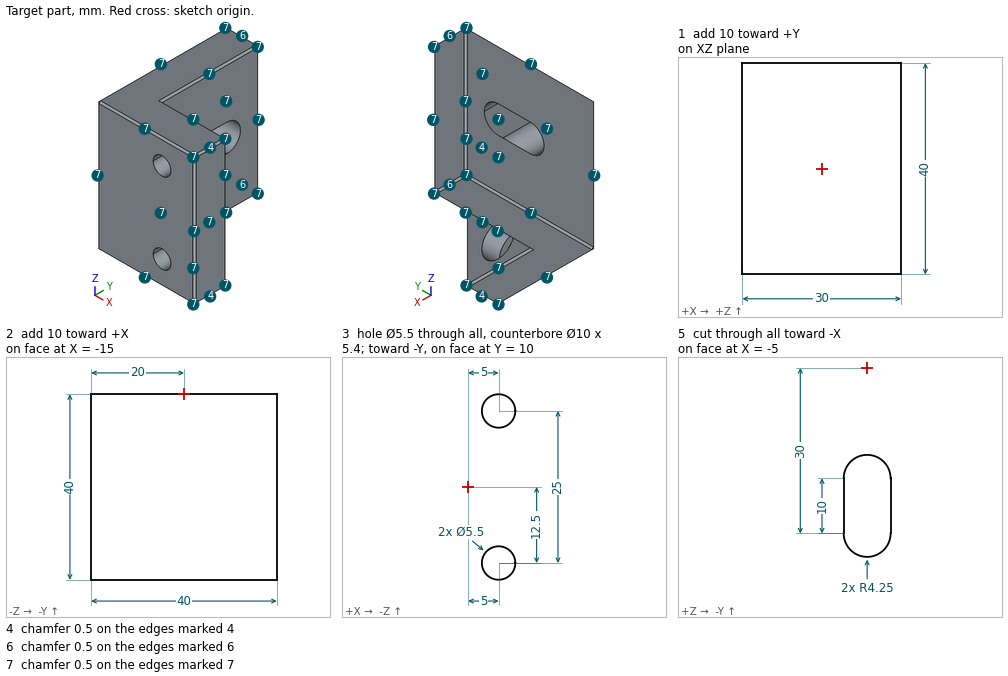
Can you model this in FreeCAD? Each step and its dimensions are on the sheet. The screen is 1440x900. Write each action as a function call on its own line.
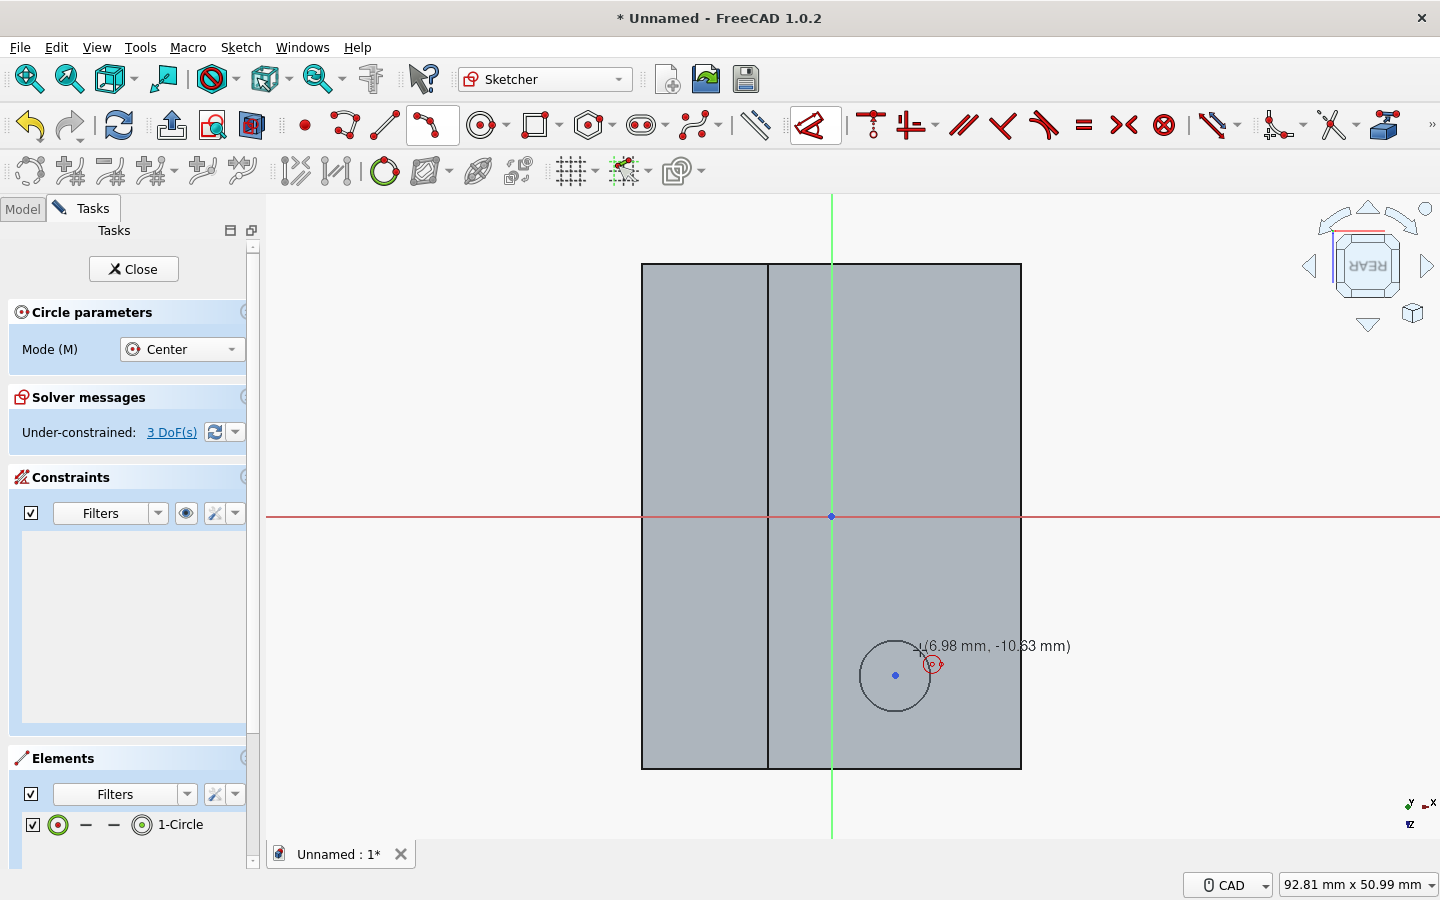
click(895, 358)
click(920, 334)
key(Escape)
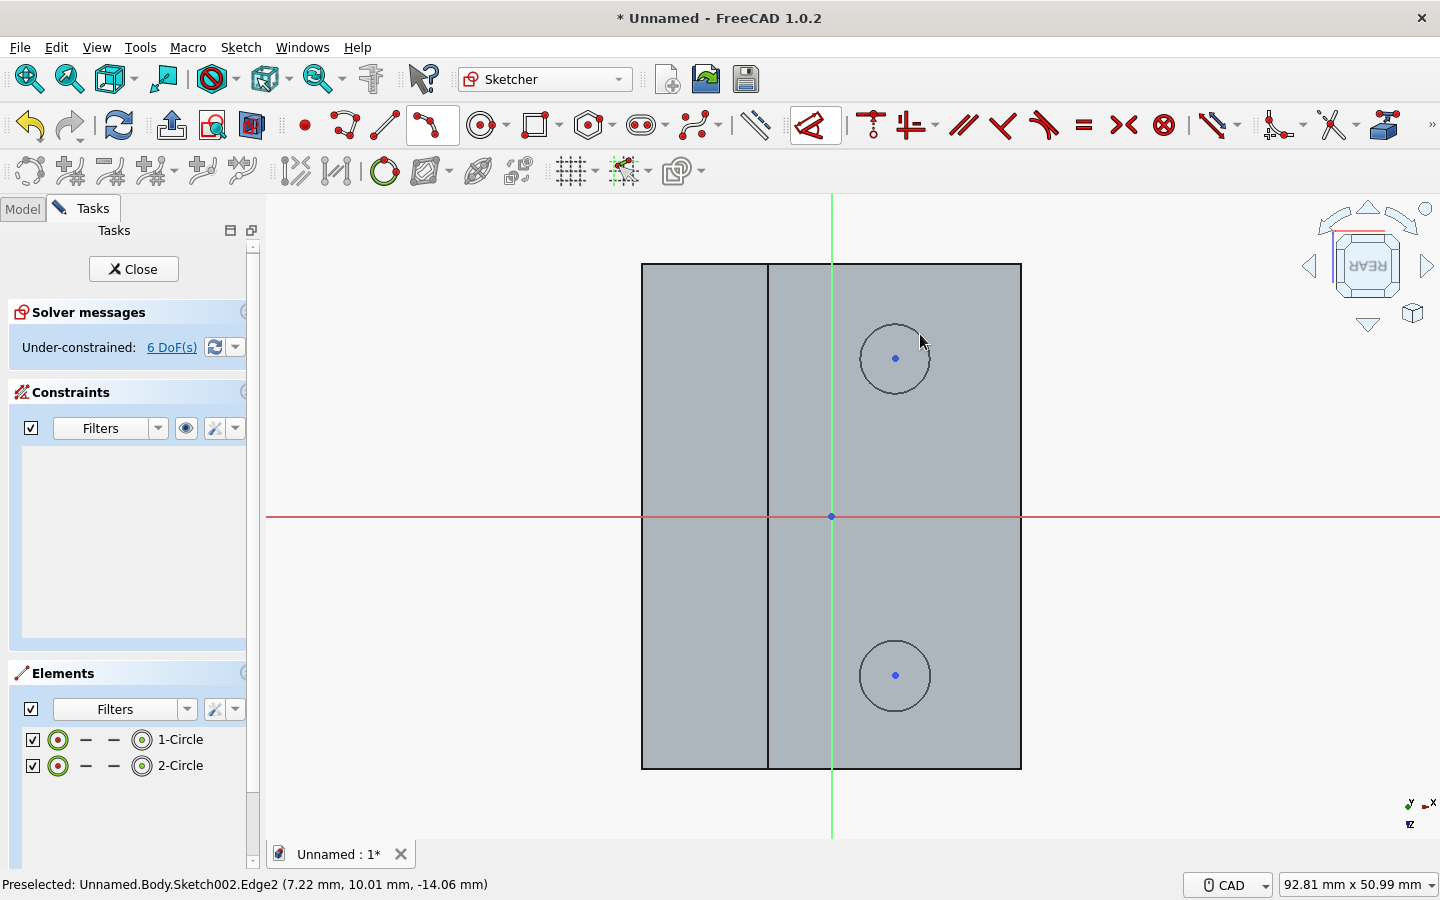
click(920, 651)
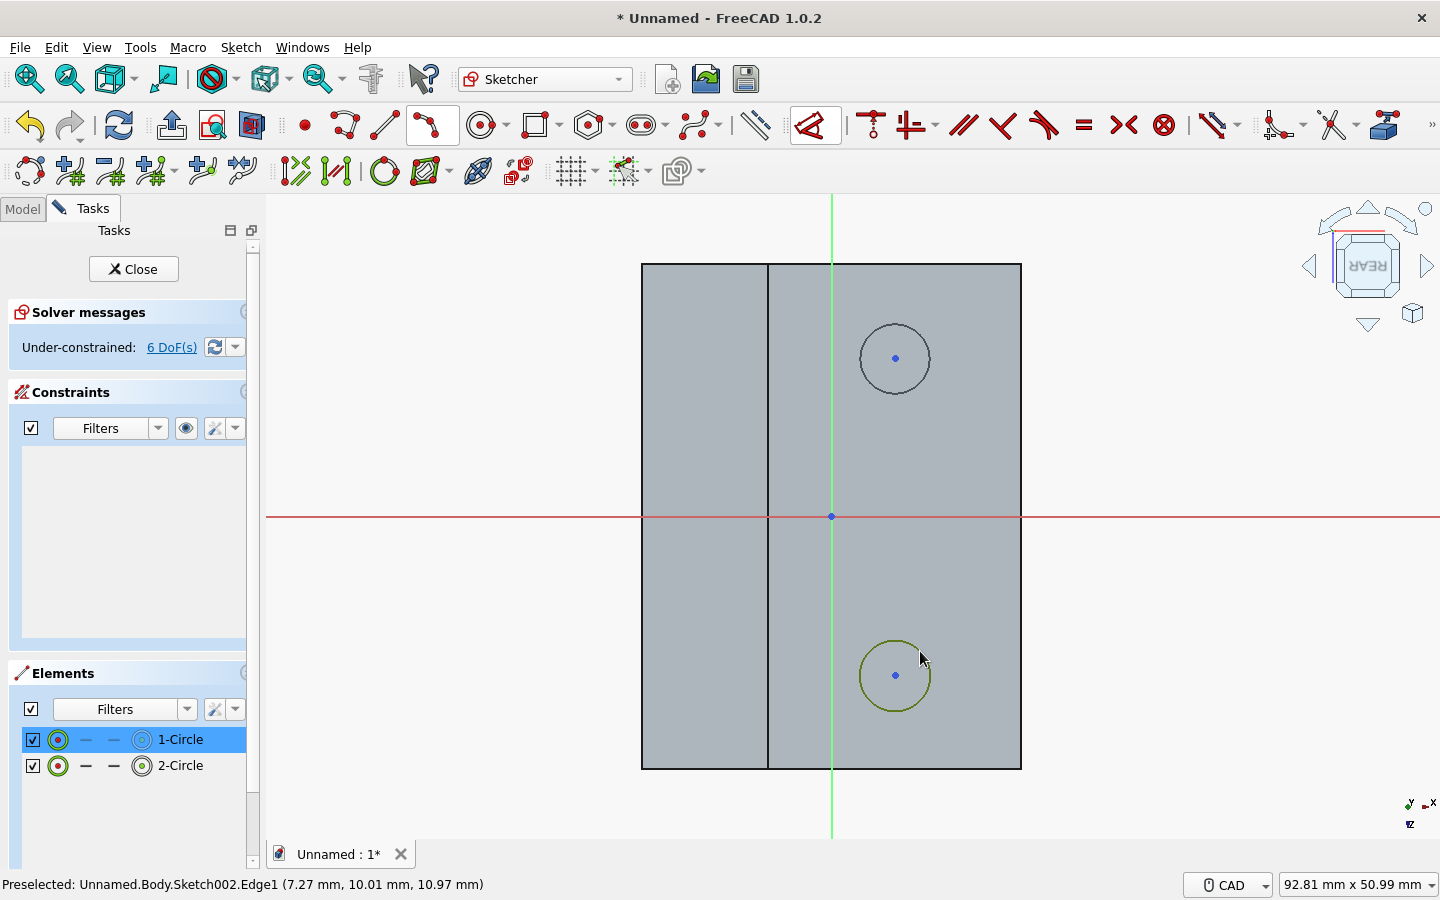
click(919, 334)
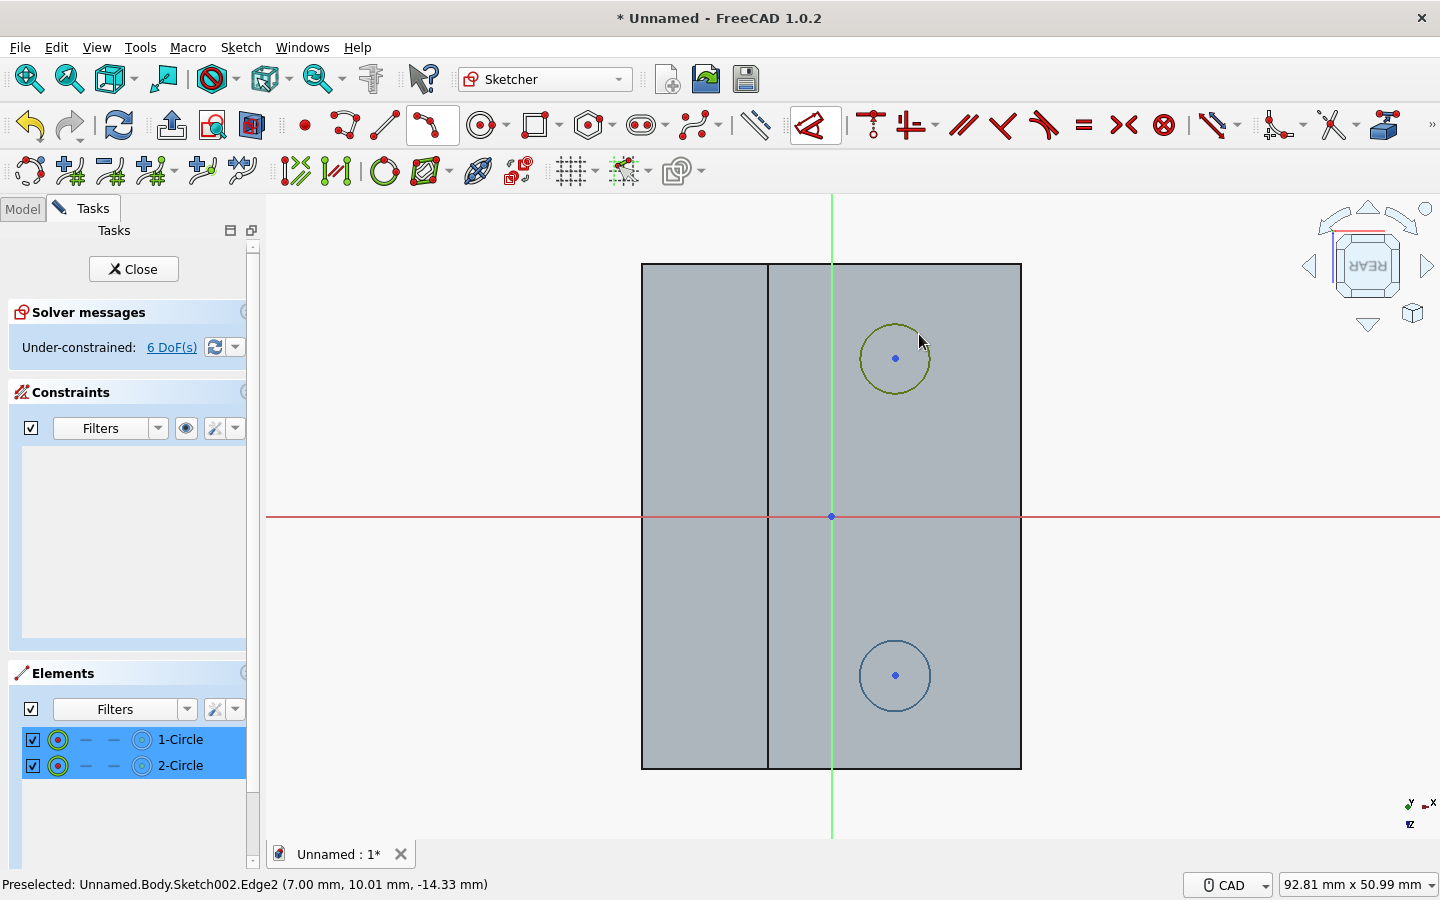
click(1084, 126)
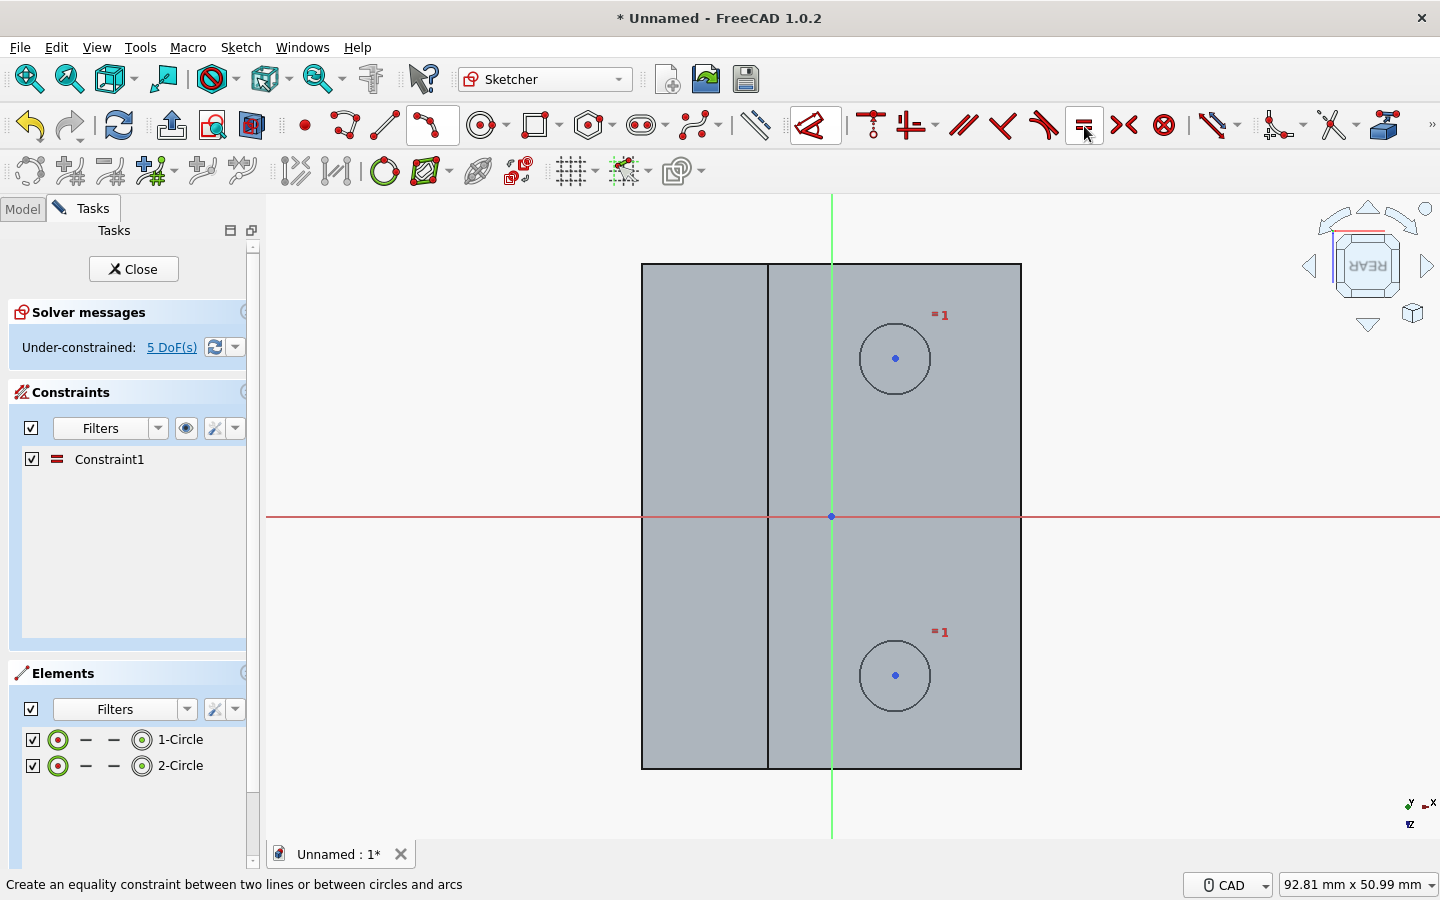
click(920, 651)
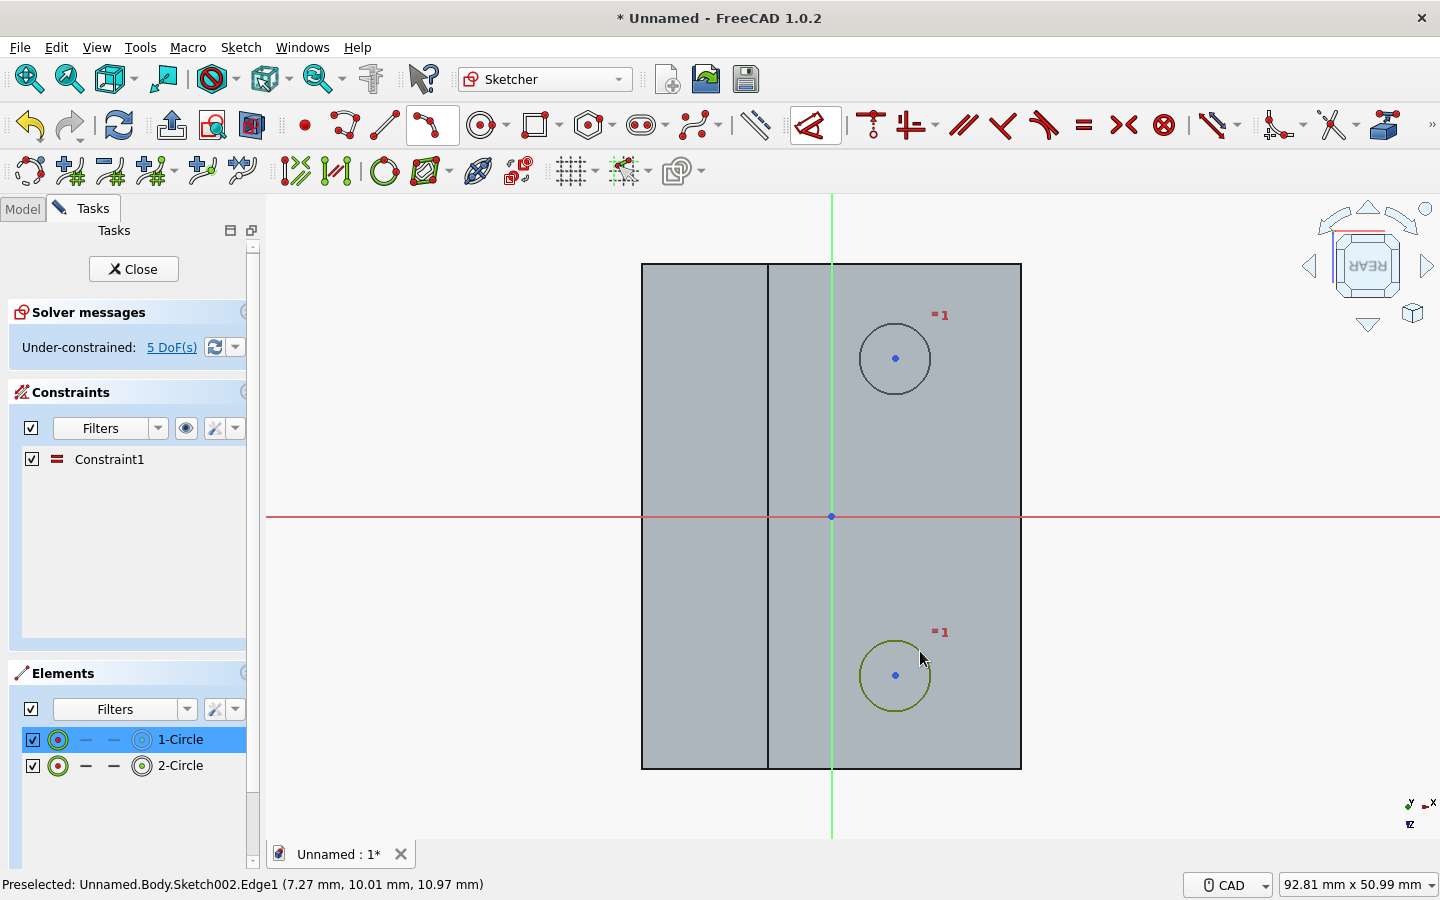
click(836, 126)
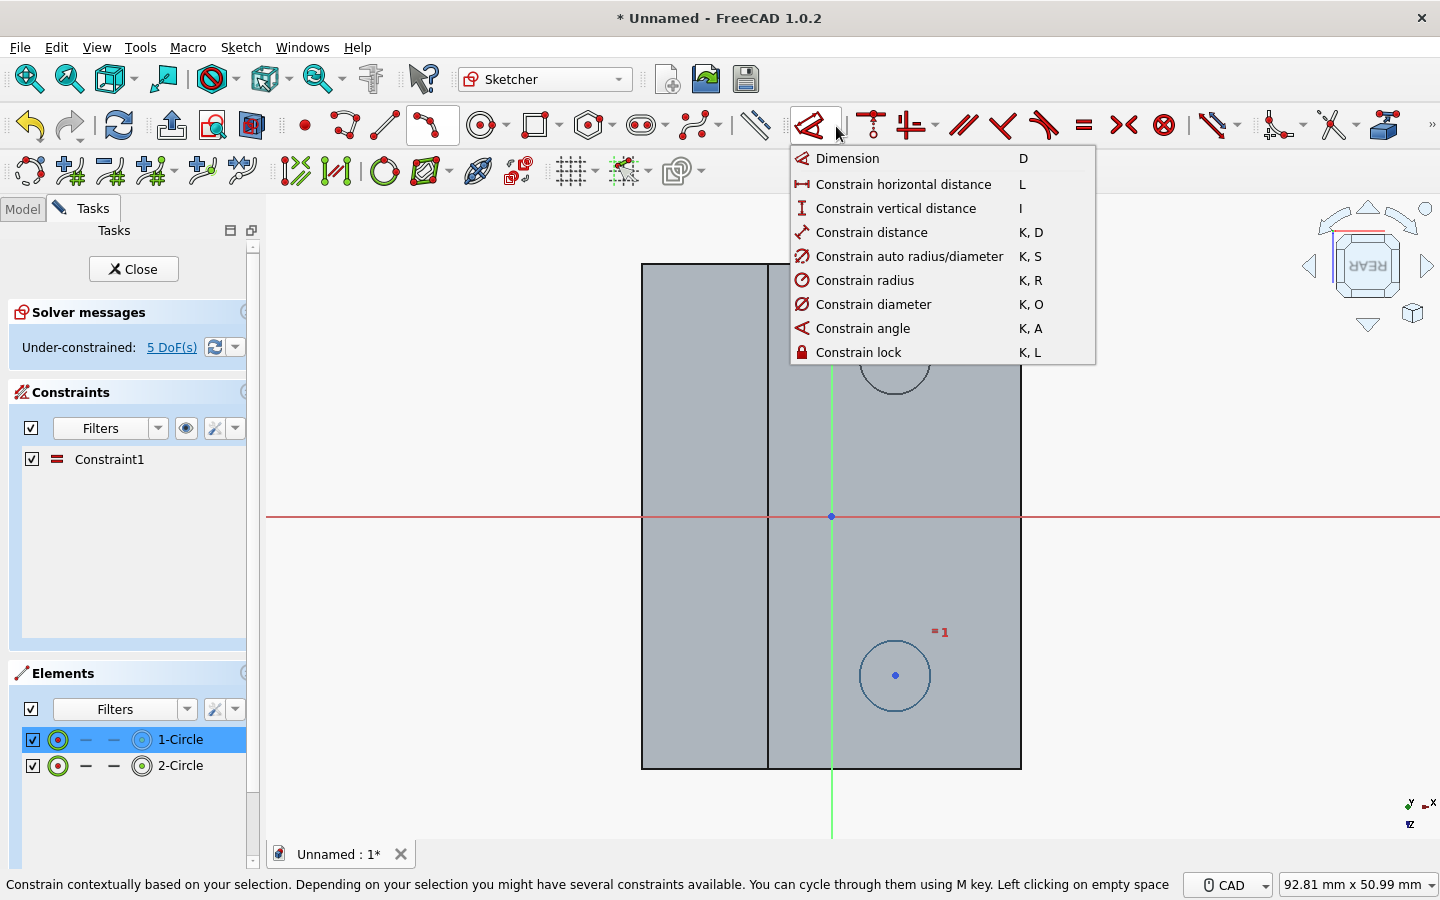
click(943, 304)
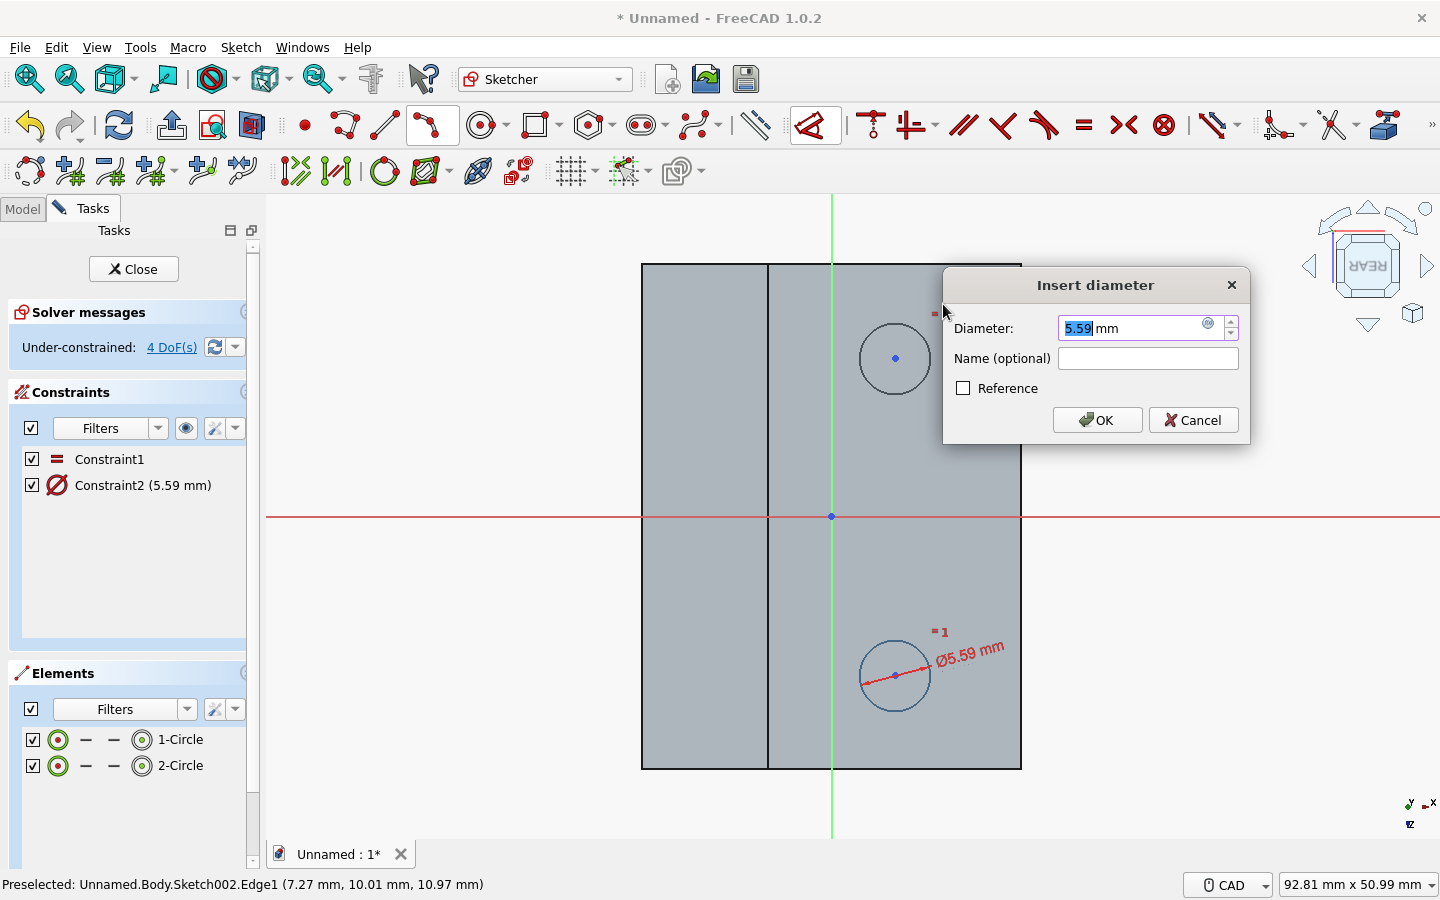
text(5.5)
key(Return)